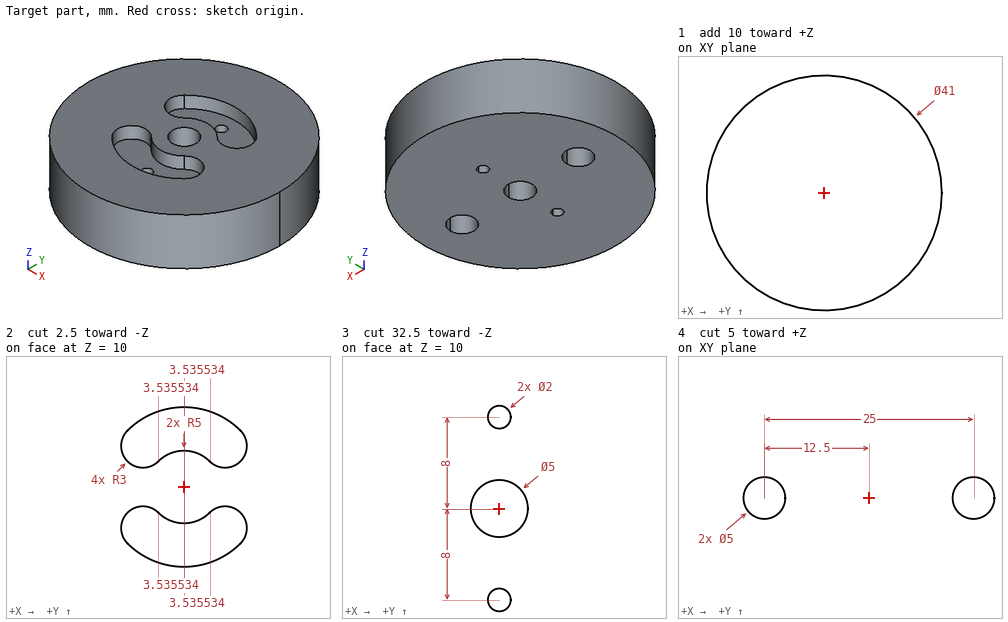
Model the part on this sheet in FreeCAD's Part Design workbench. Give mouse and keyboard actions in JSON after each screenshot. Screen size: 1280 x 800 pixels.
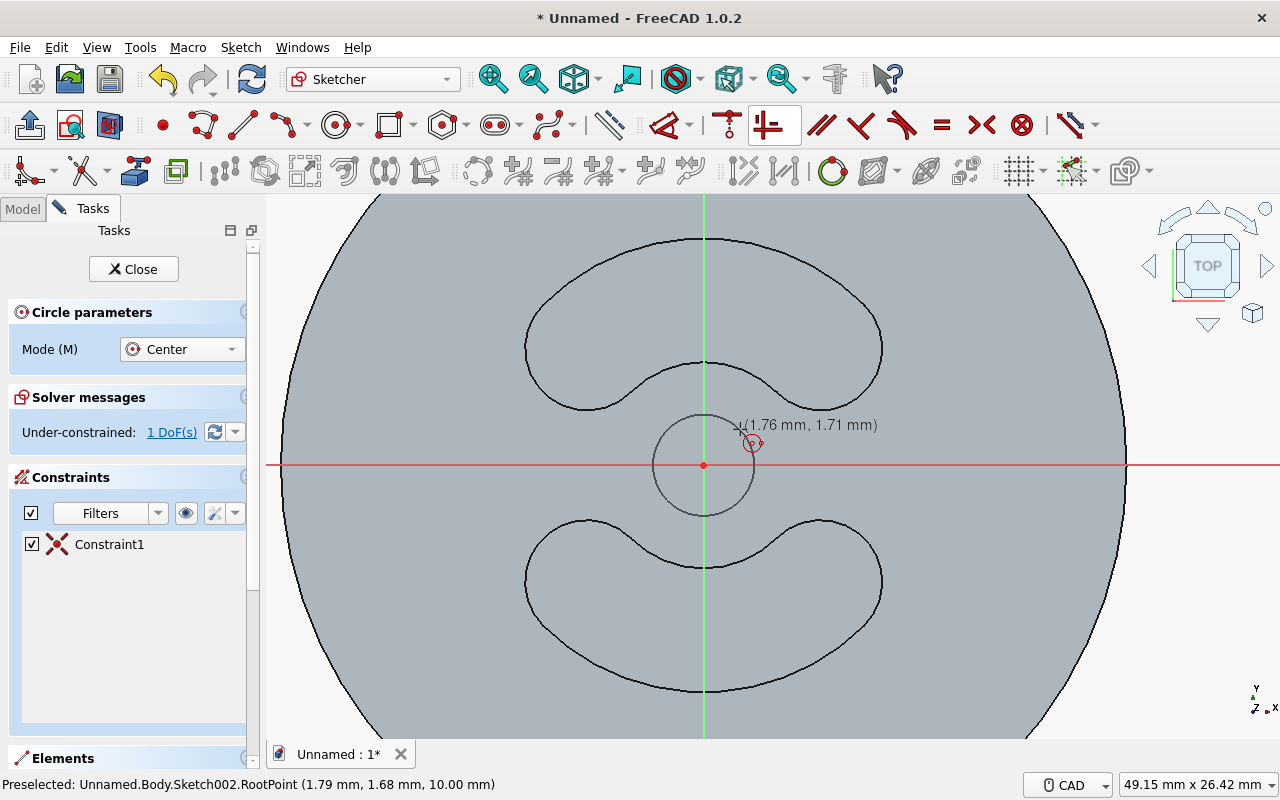
{"action": "left_click", "coordinate": [704, 300]}
{"action": "left_click", "coordinate": [718, 286]}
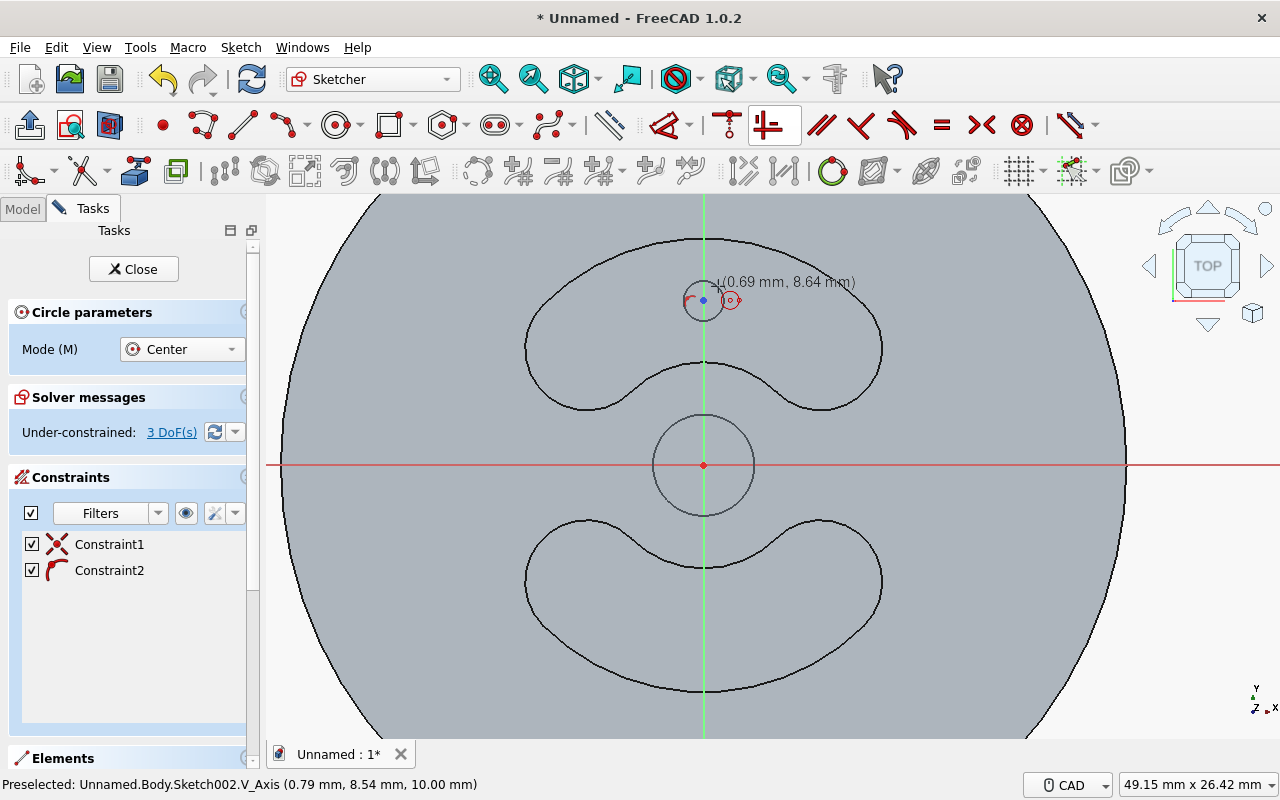
{"action": "left_click", "coordinate": [704, 630]}
{"action": "left_click", "coordinate": [718, 616]}
{"action": "key", "text": "Escape"}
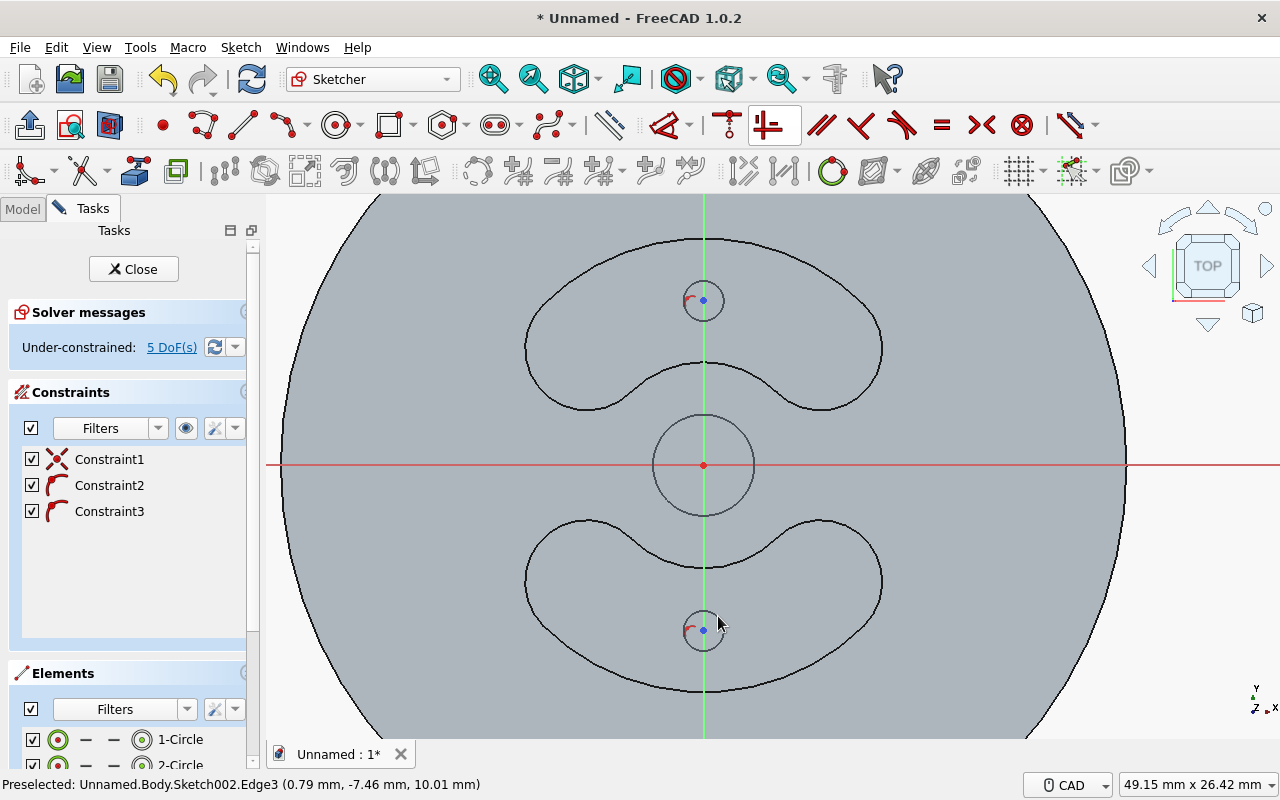
{"action": "left_click", "coordinate": [718, 287]}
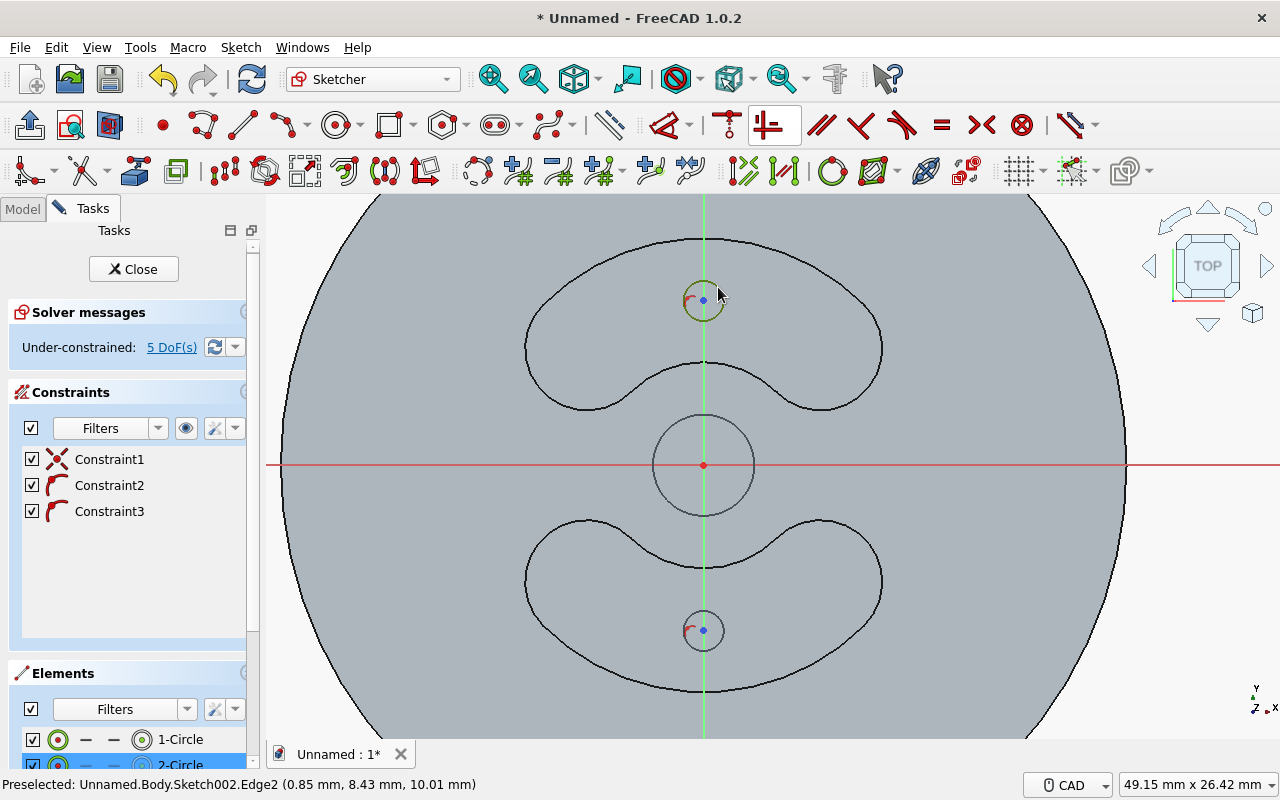
{"action": "left_click", "coordinate": [718, 617]}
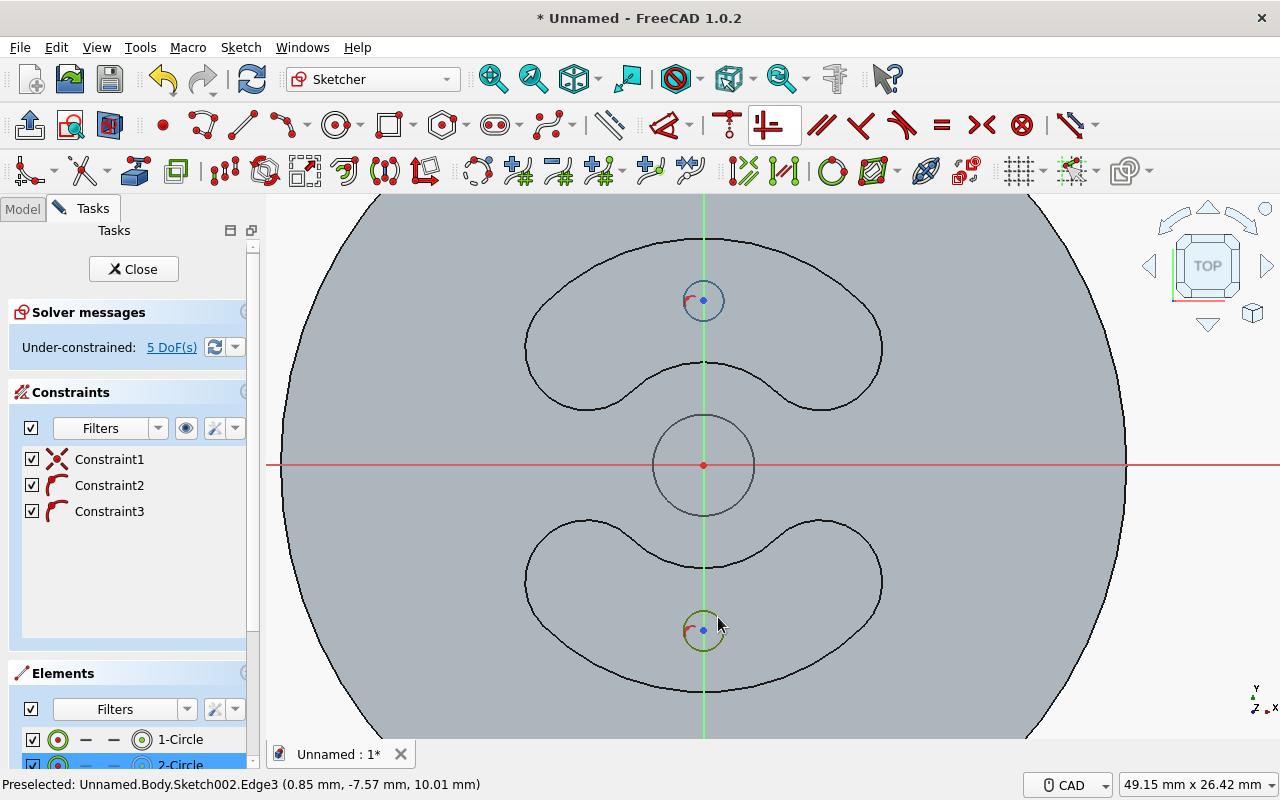
{"action": "left_click", "coordinate": [942, 126]}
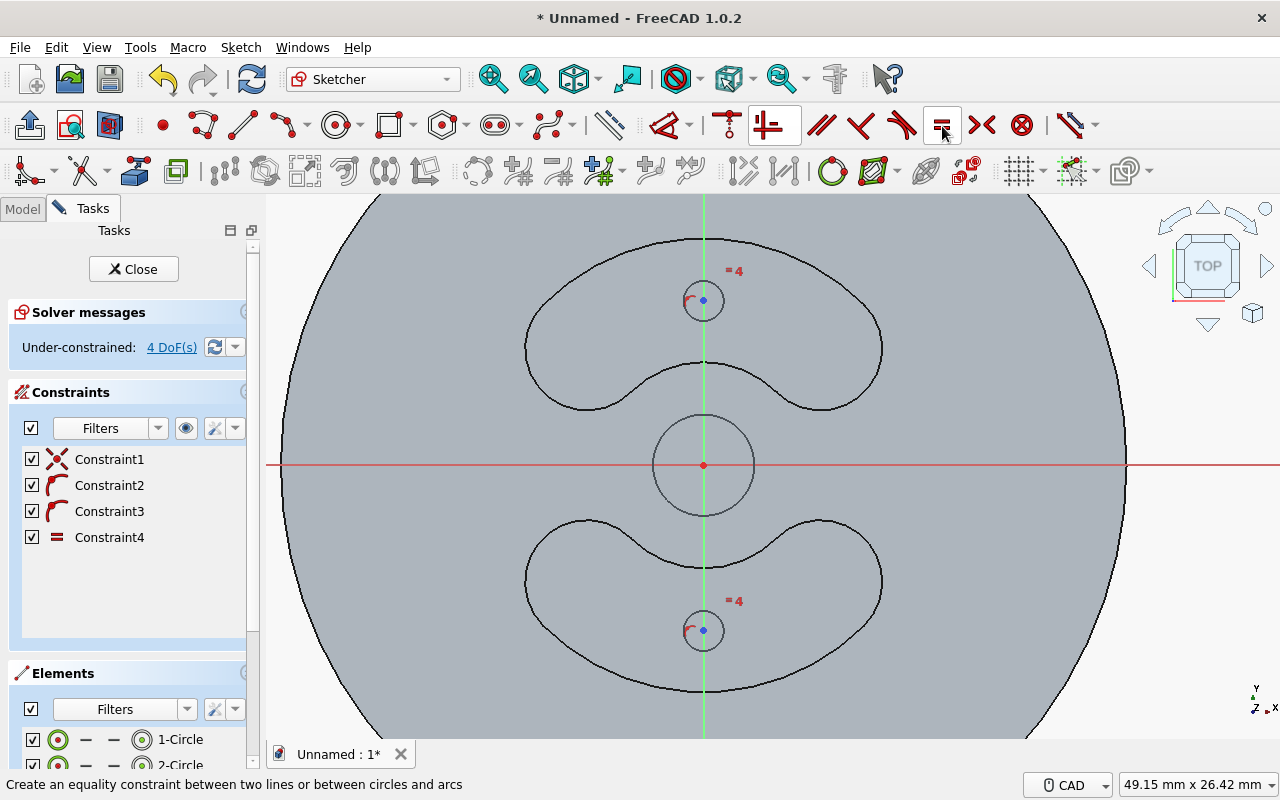
{"action": "key", "text": "d"}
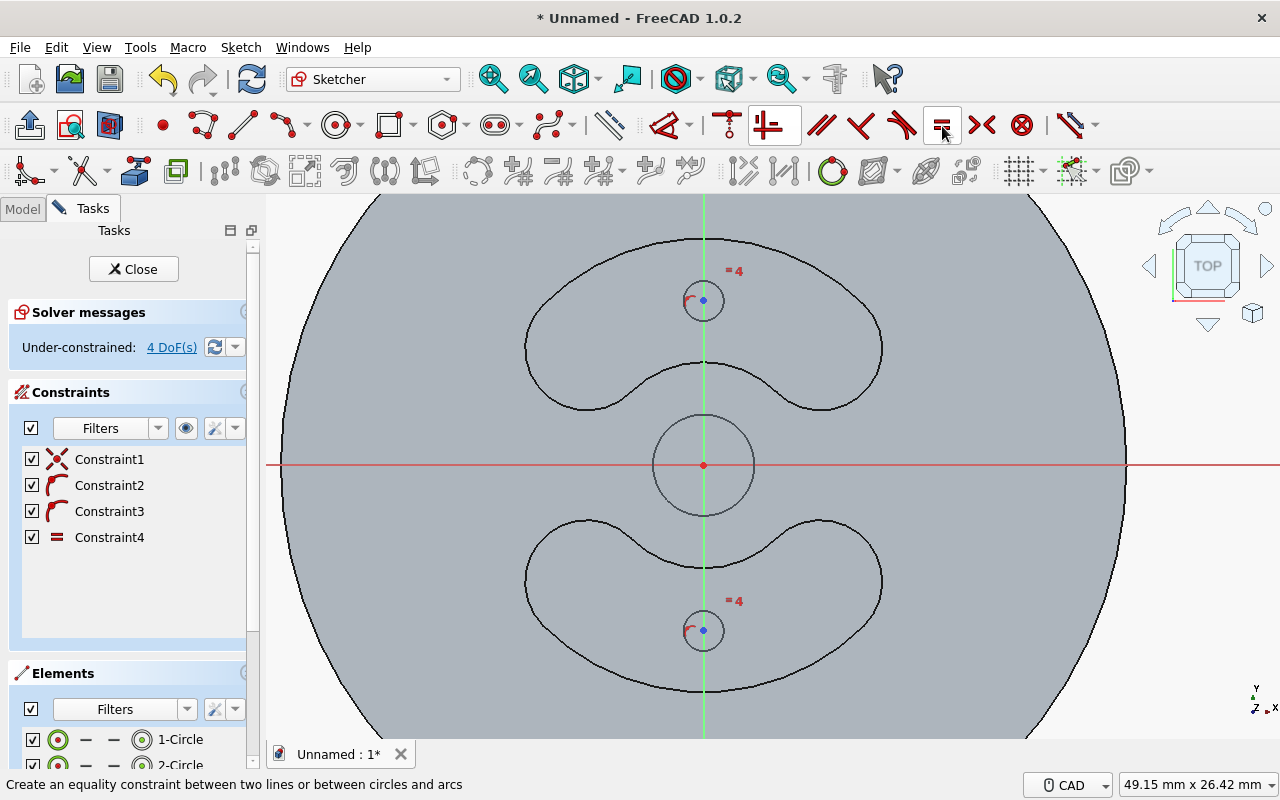
{"action": "left_click", "coordinate": [739, 429]}
{"action": "left_click", "coordinate": [761, 406]}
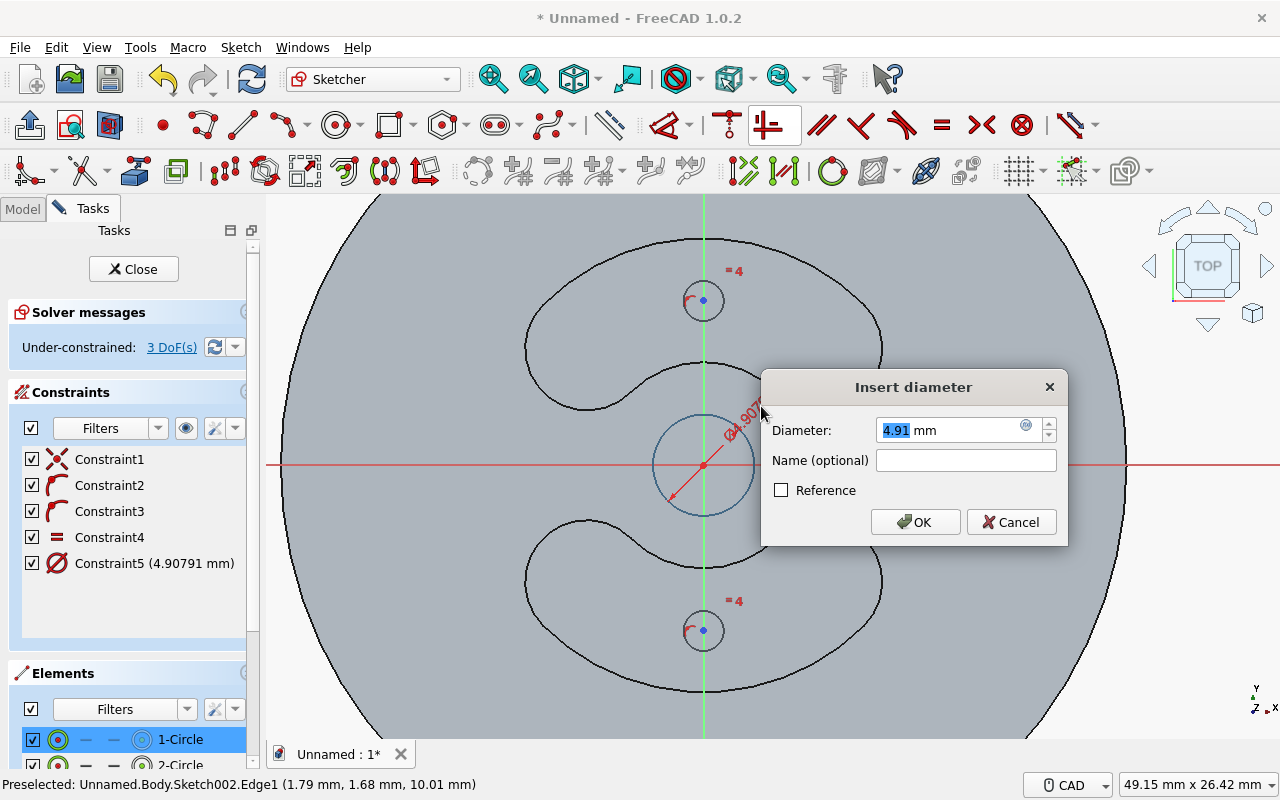
{"action": "type", "text": "5"}
{"action": "key", "text": "Return"}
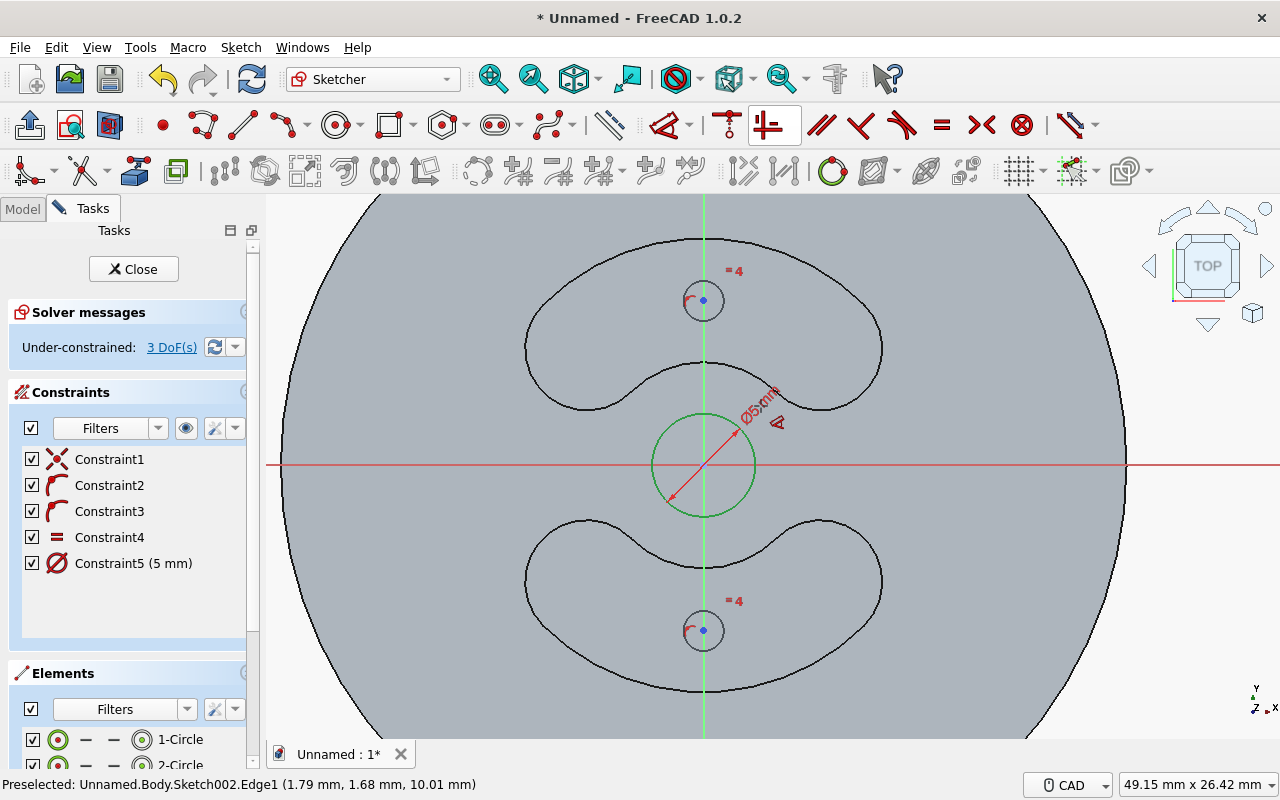
{"action": "left_click", "coordinate": [718, 287]}
{"action": "left_click", "coordinate": [741, 265]}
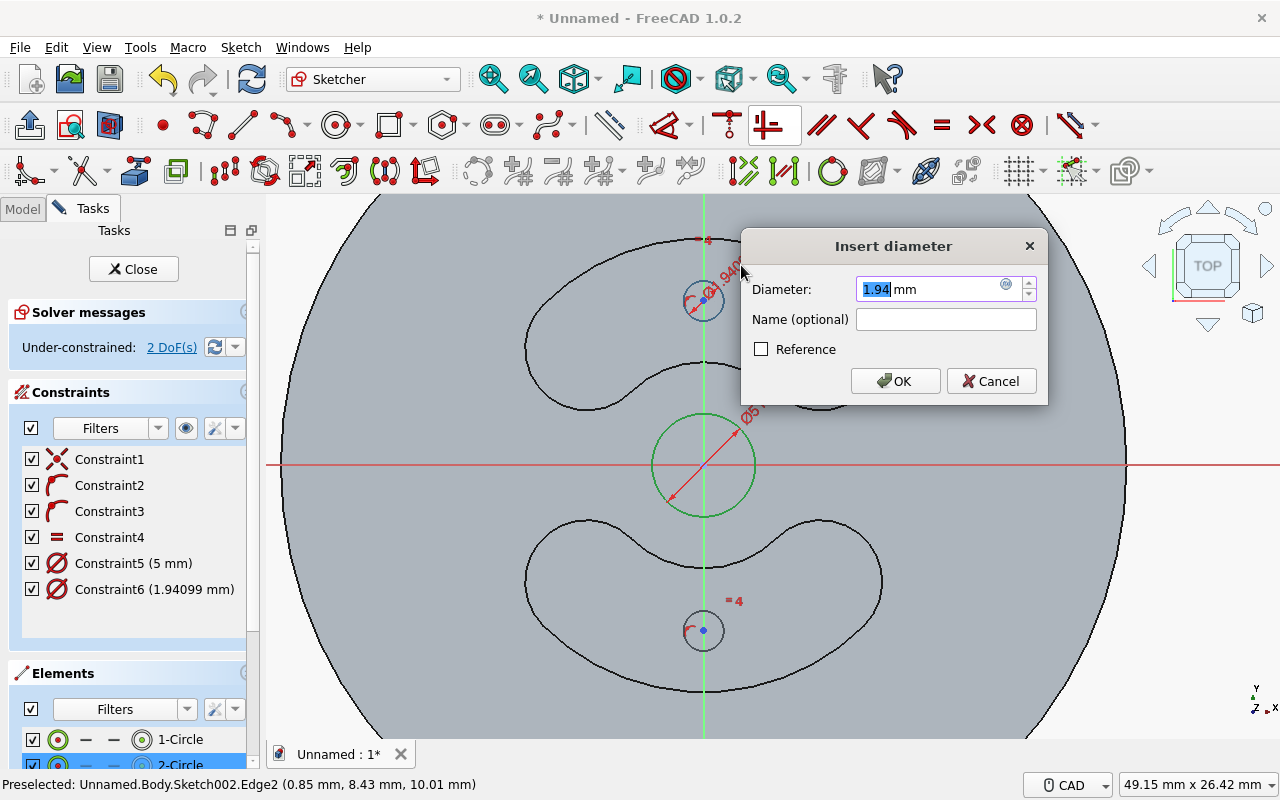
{"action": "type", "text": "2"}
{"action": "key", "text": "Return"}